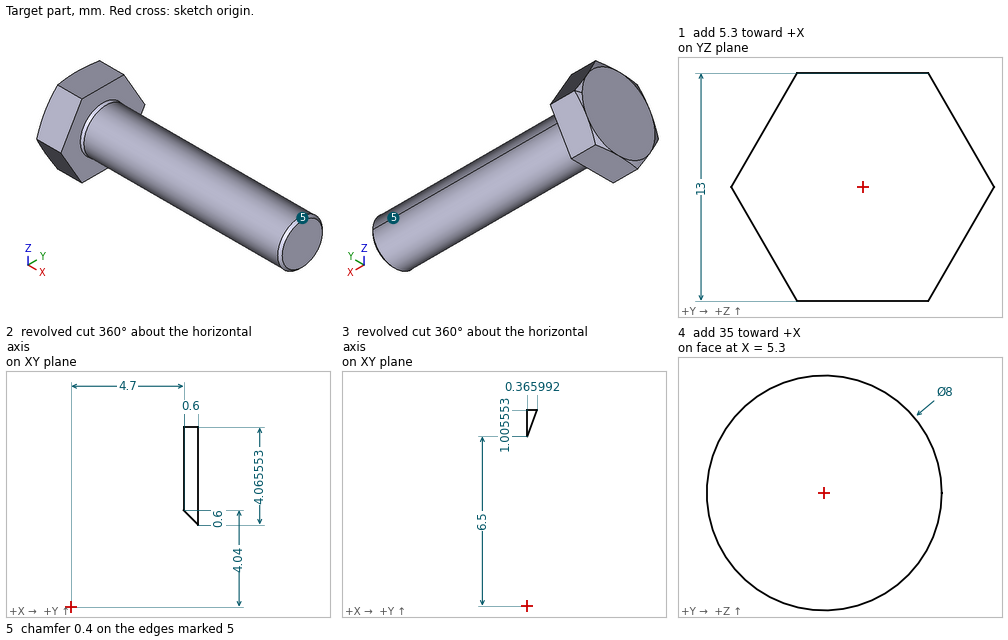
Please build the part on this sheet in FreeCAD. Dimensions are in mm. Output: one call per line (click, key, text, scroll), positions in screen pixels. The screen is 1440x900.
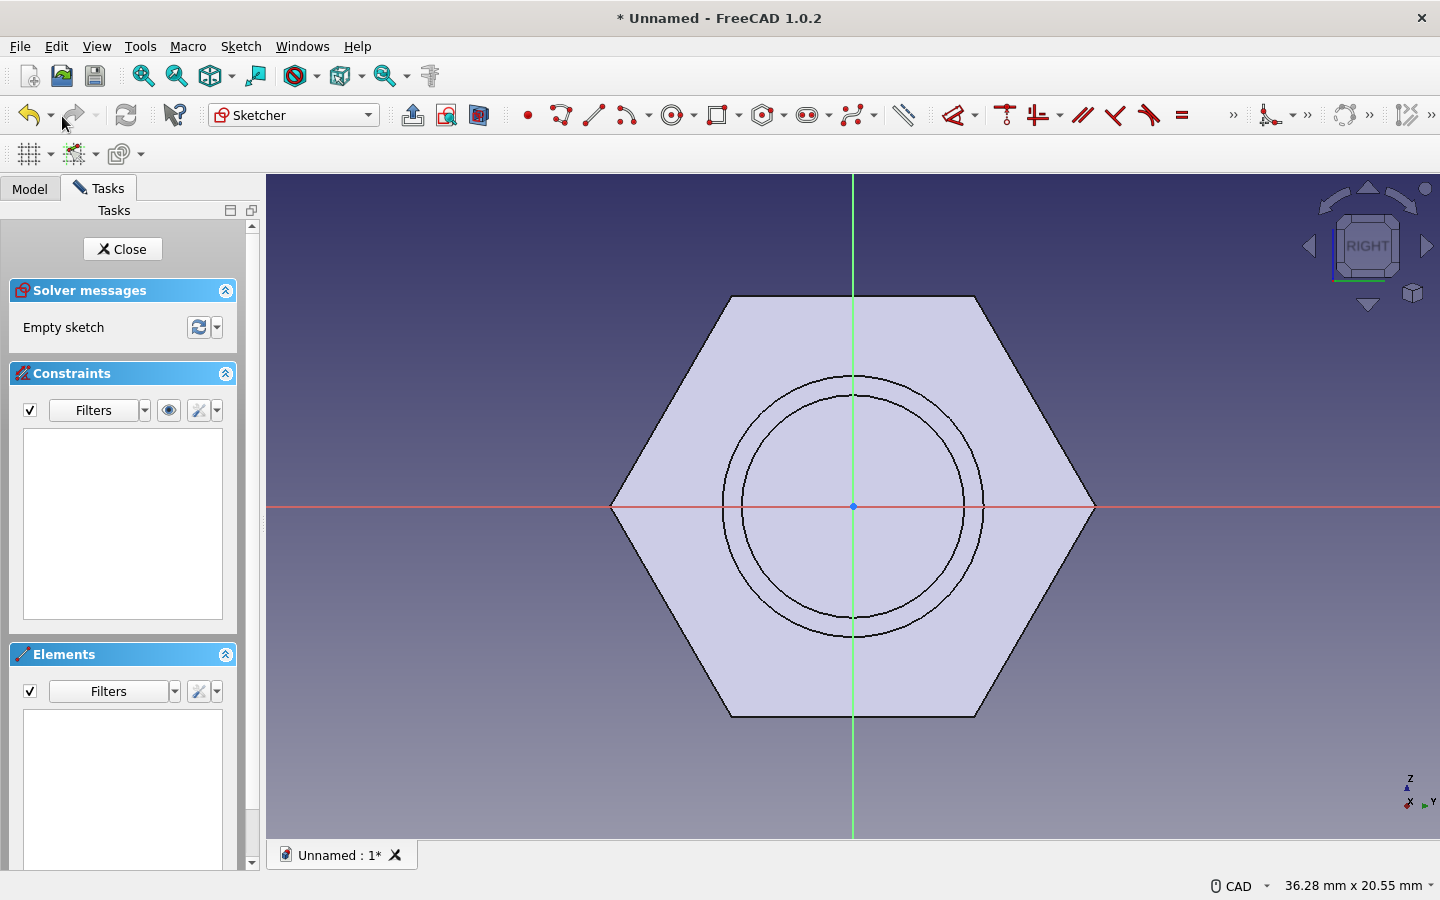
scroll(936, 506, up, 3)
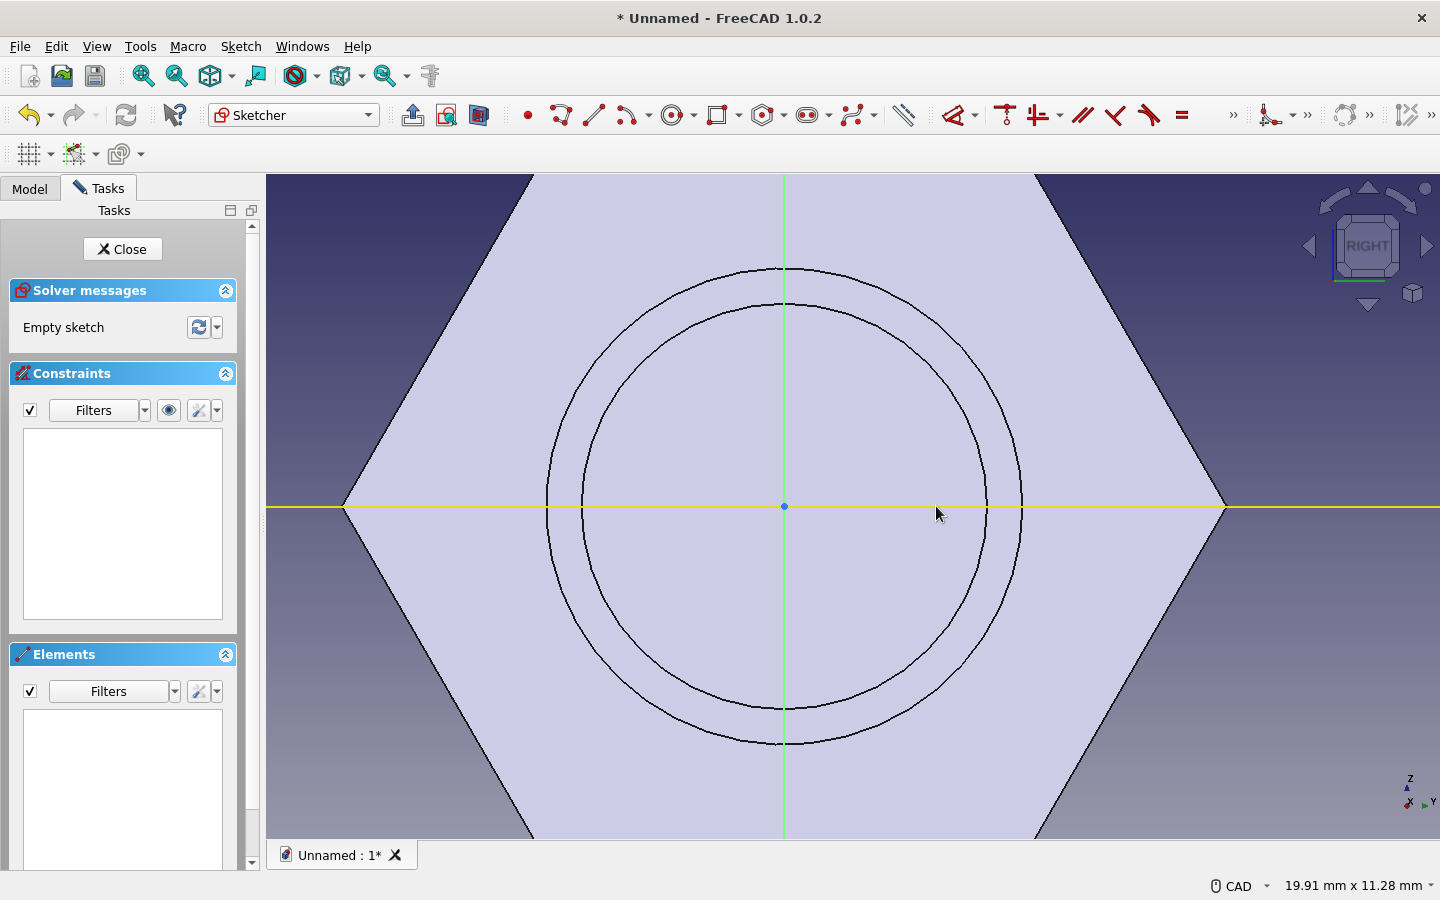
click(672, 116)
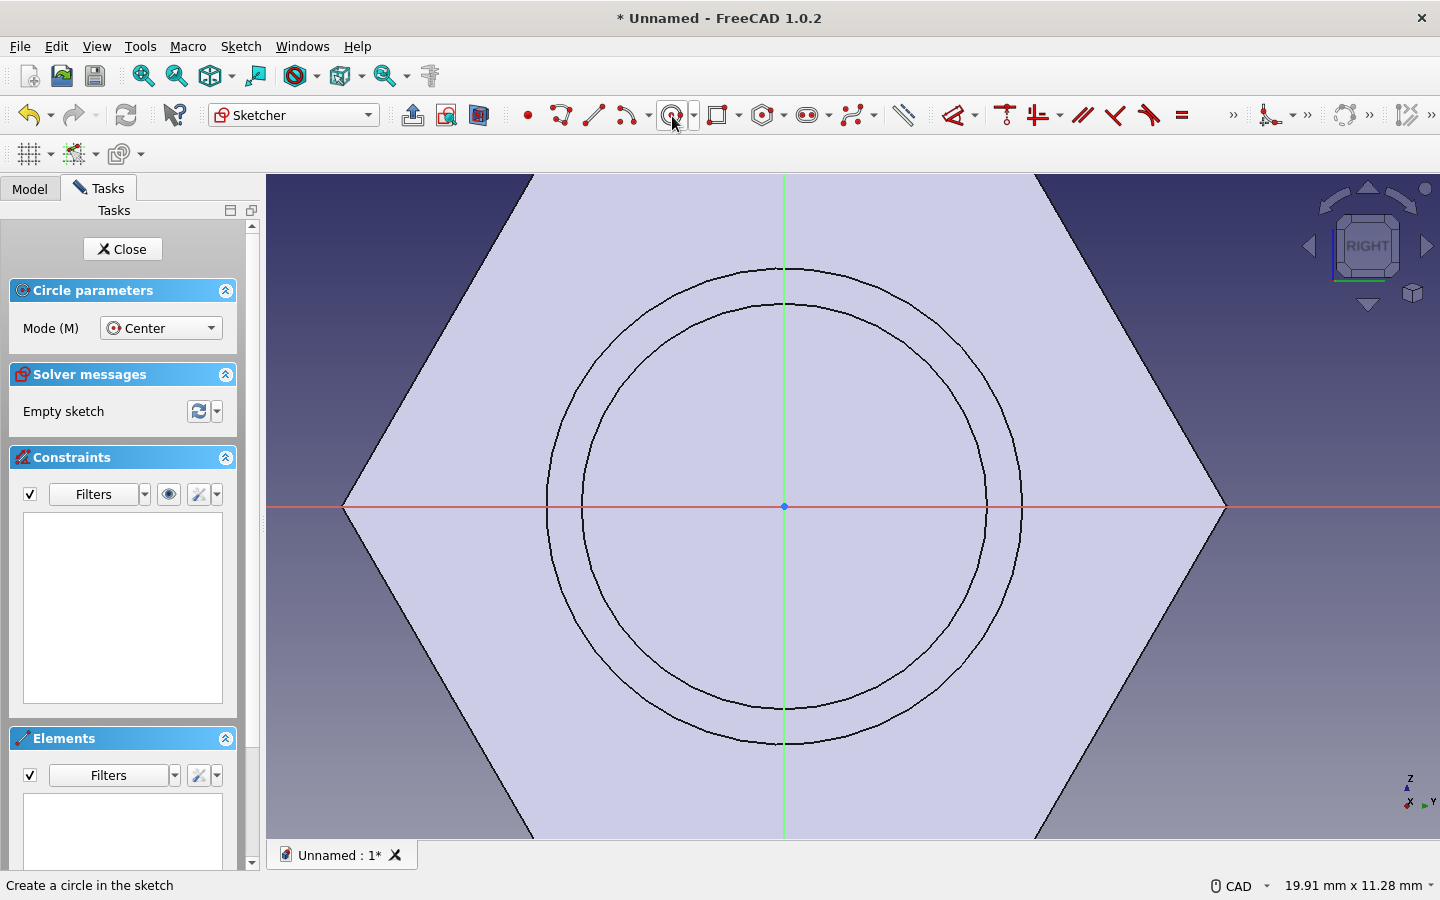
click(784, 506)
move(951, 340)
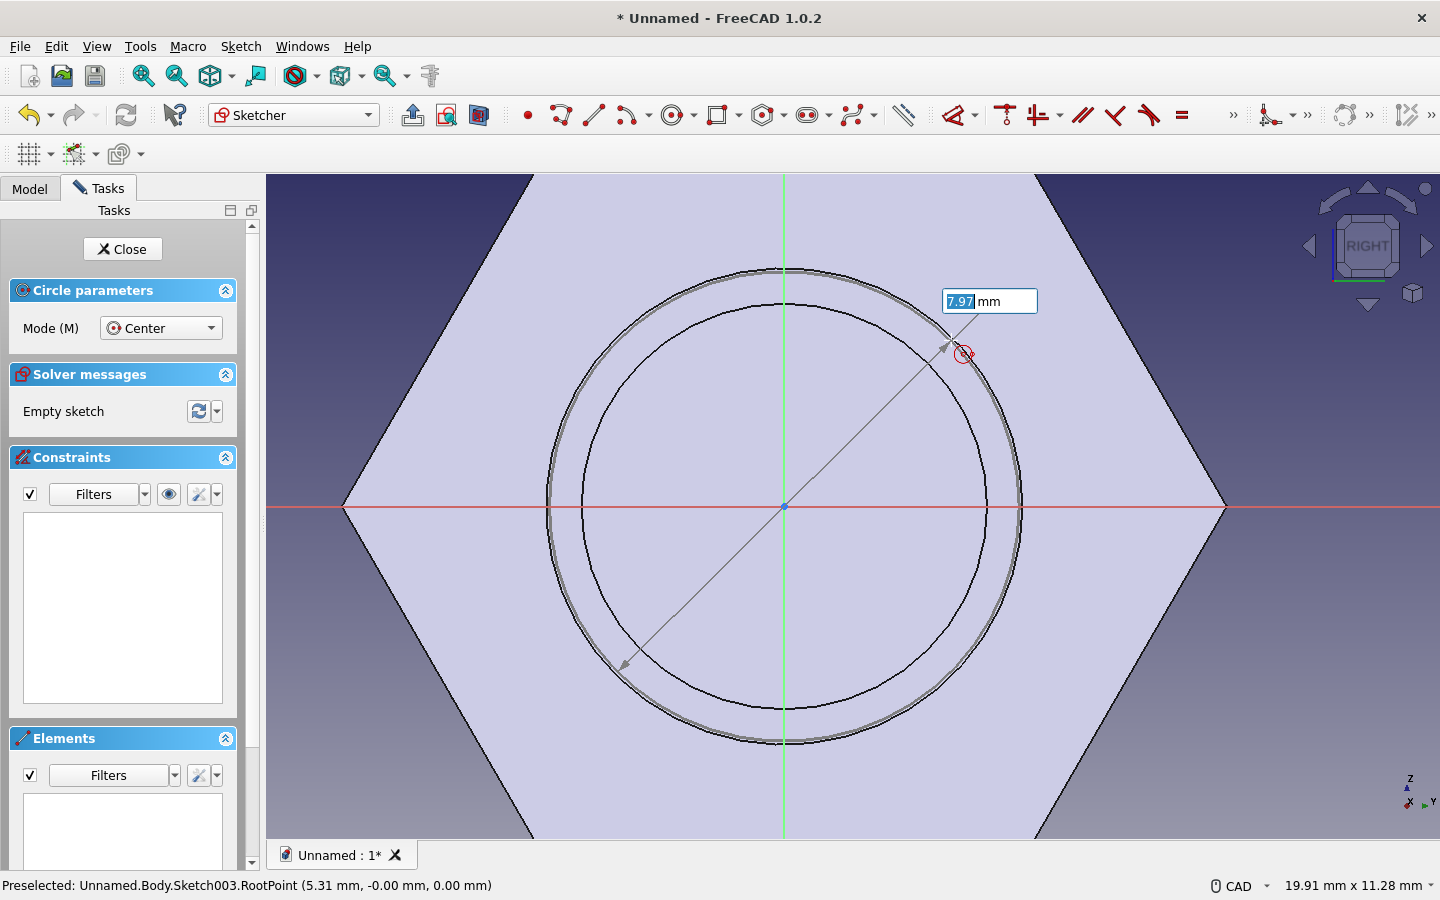
text(8)
key(Return)
key(Escape)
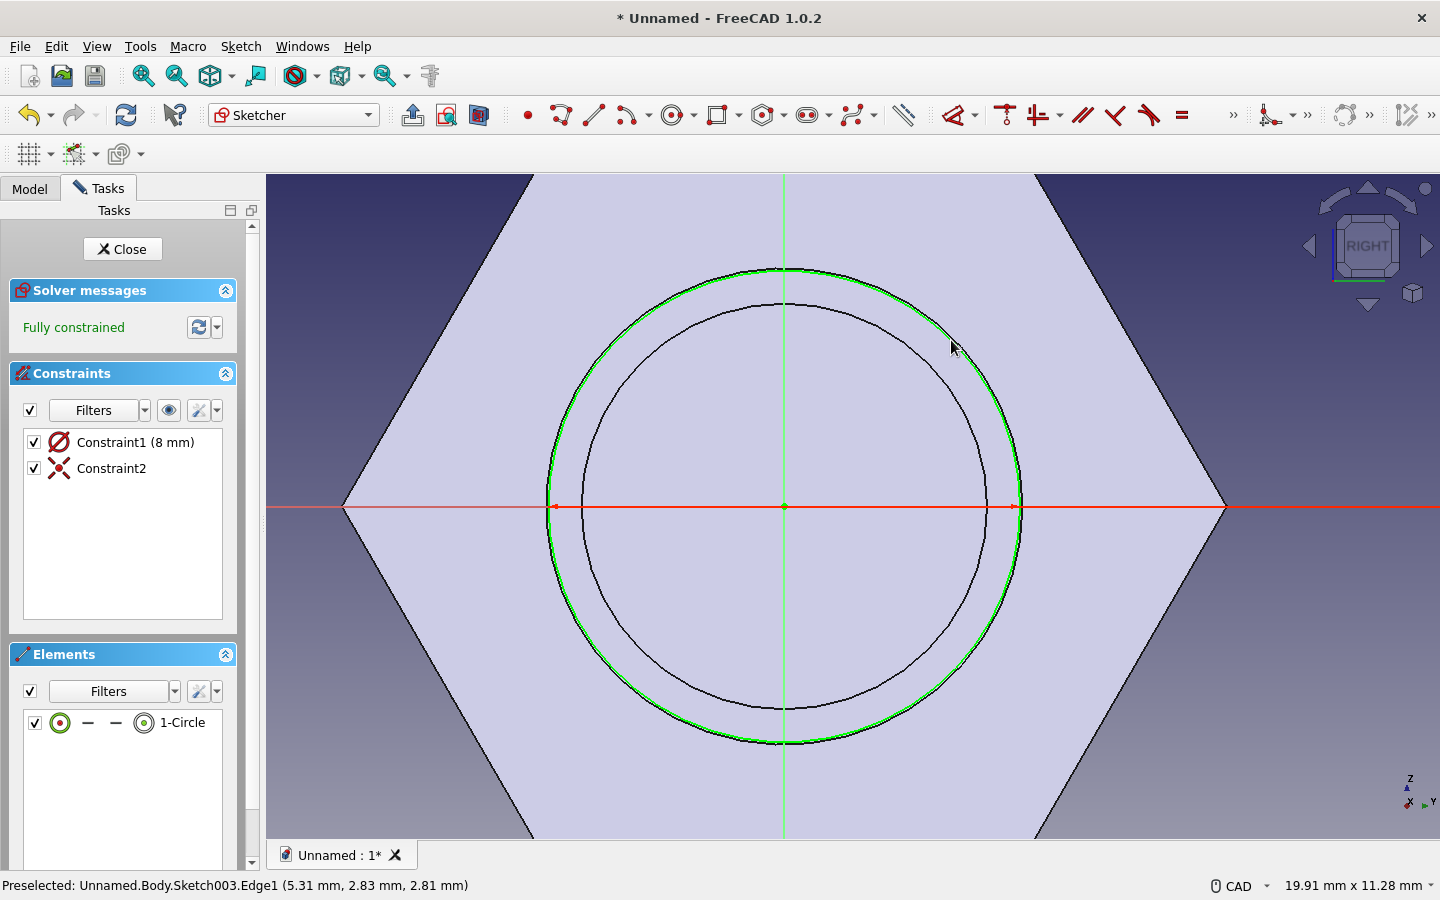
click(123, 249)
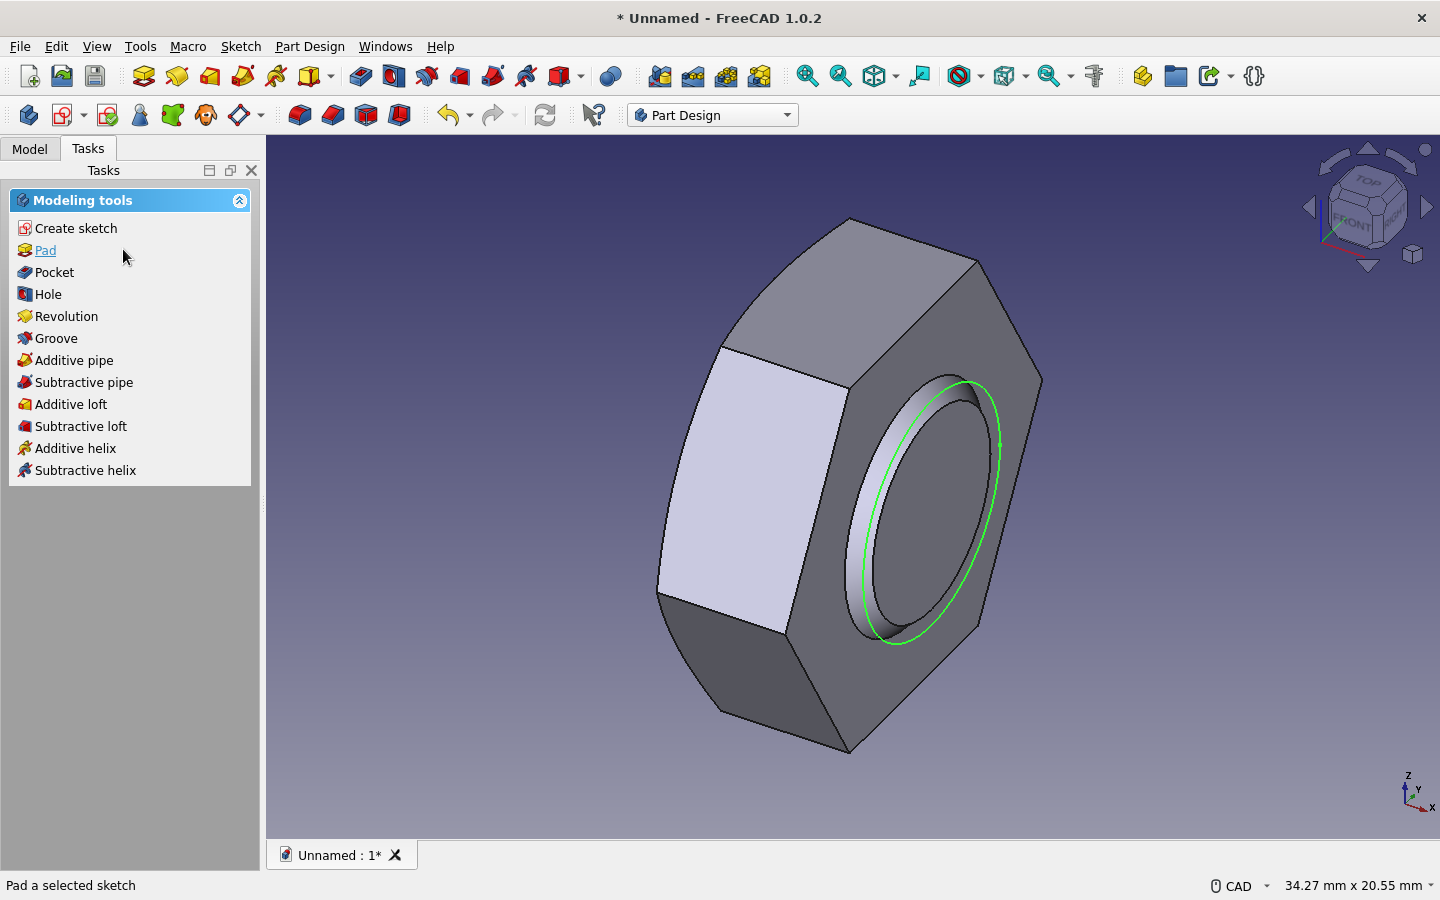
click(144, 76)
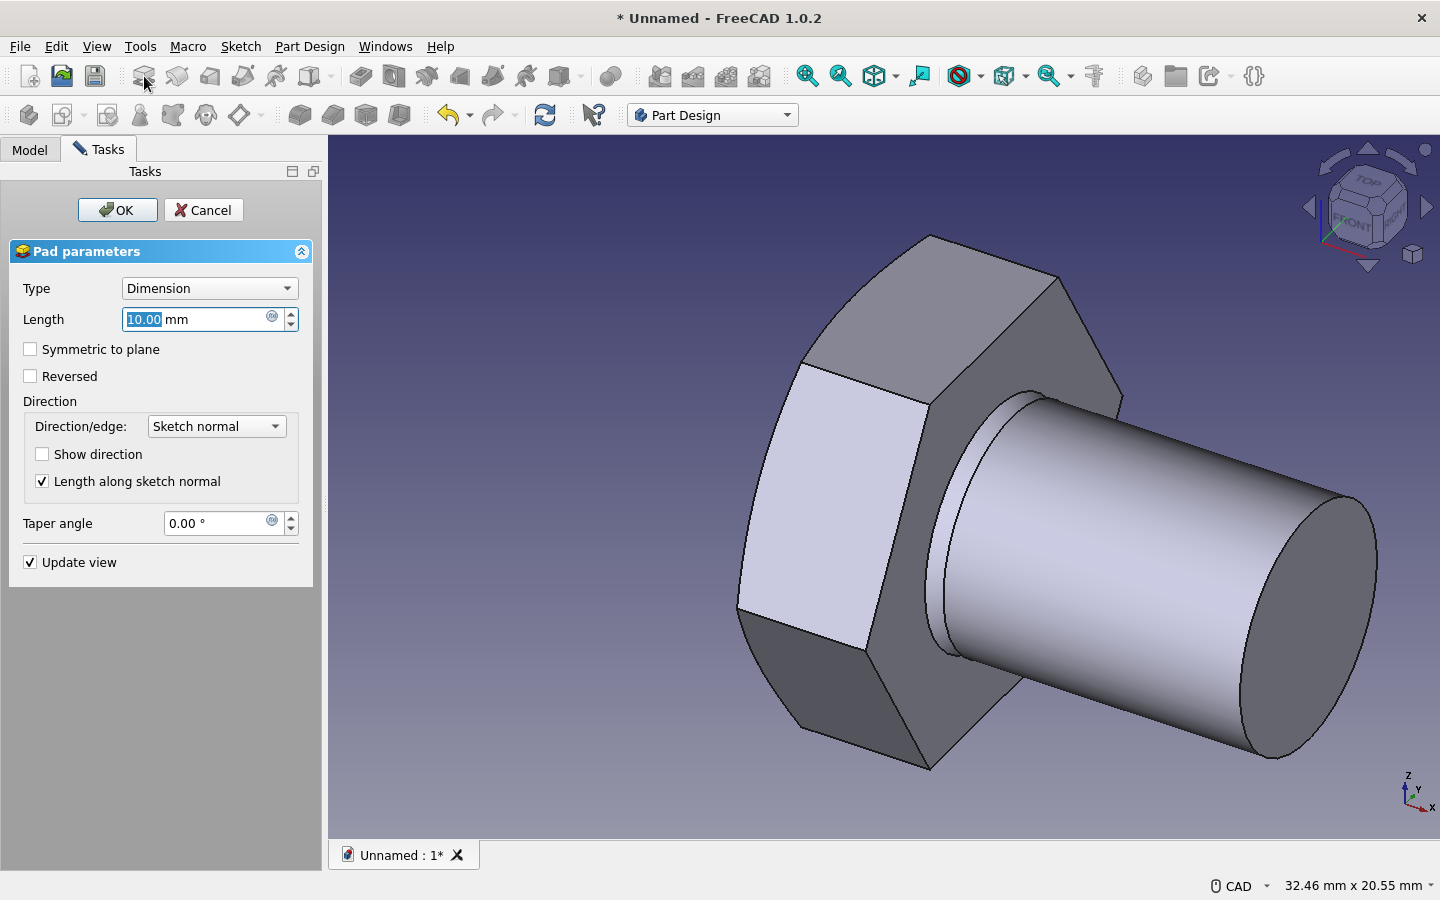
text(35)
key(Tab)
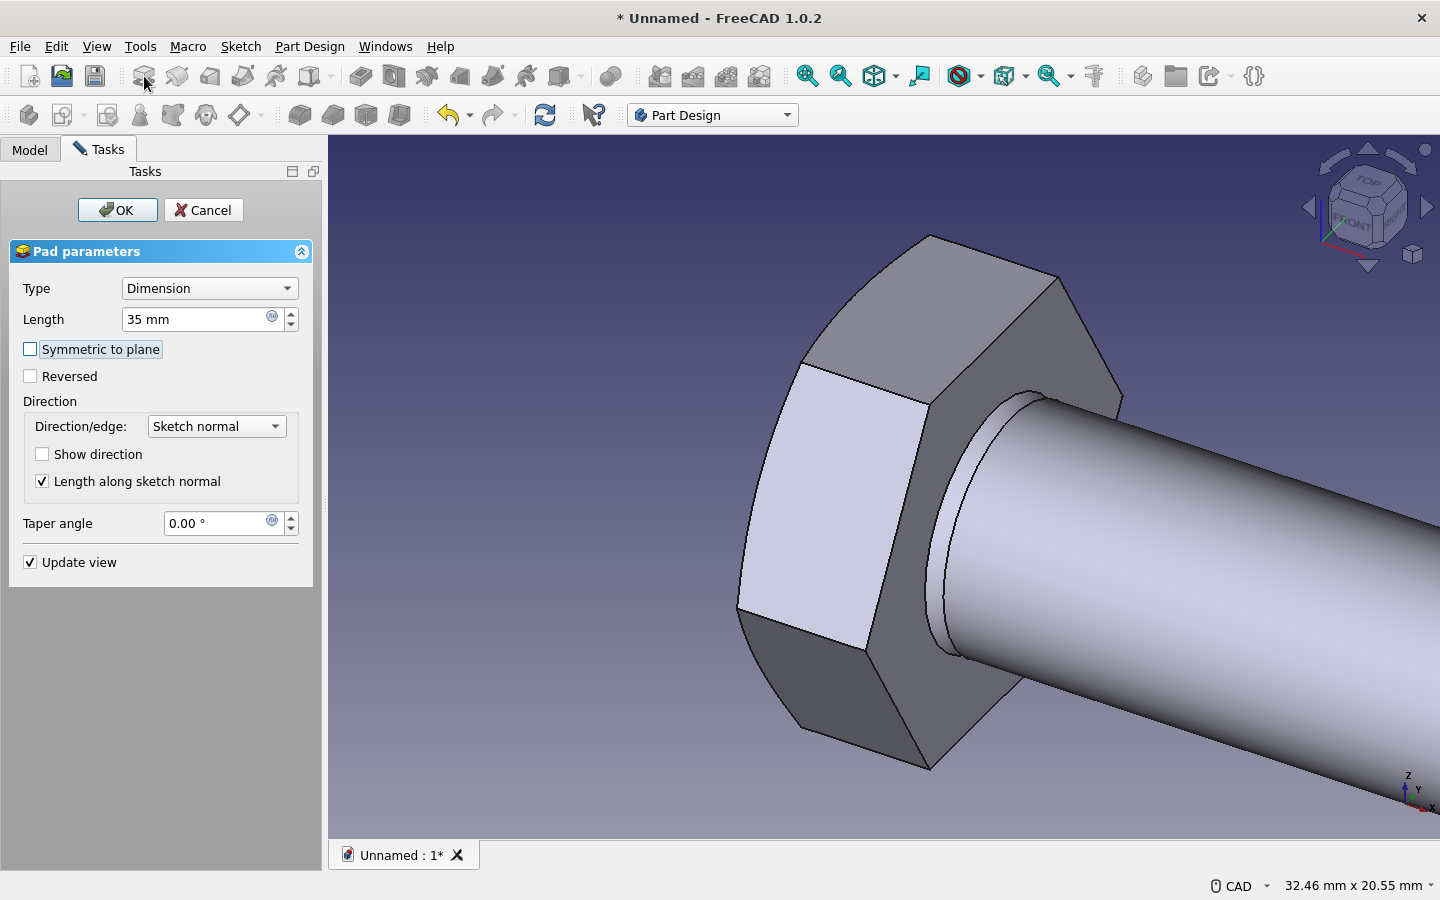
click(118, 210)